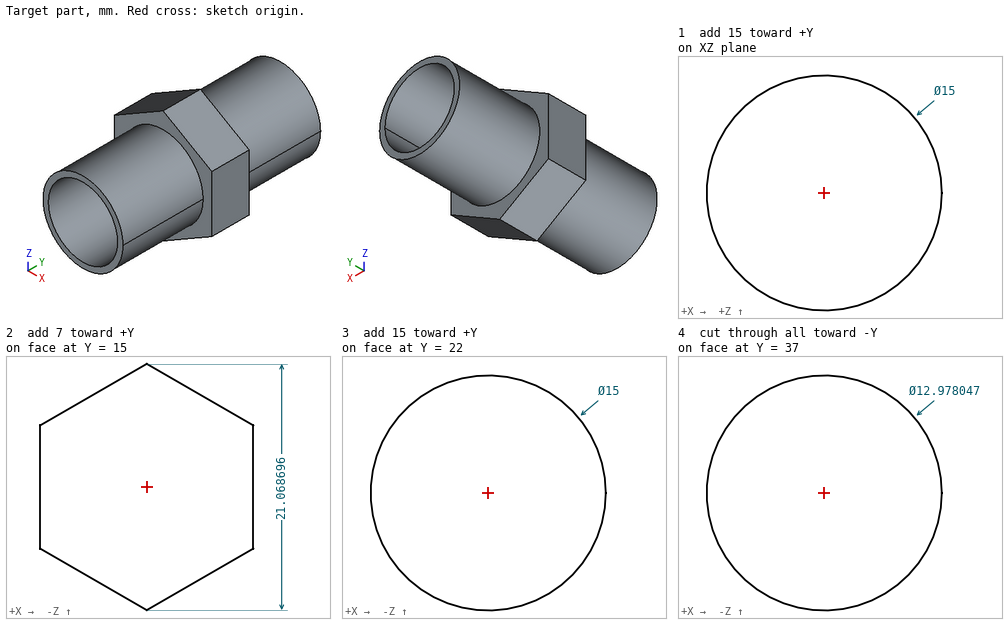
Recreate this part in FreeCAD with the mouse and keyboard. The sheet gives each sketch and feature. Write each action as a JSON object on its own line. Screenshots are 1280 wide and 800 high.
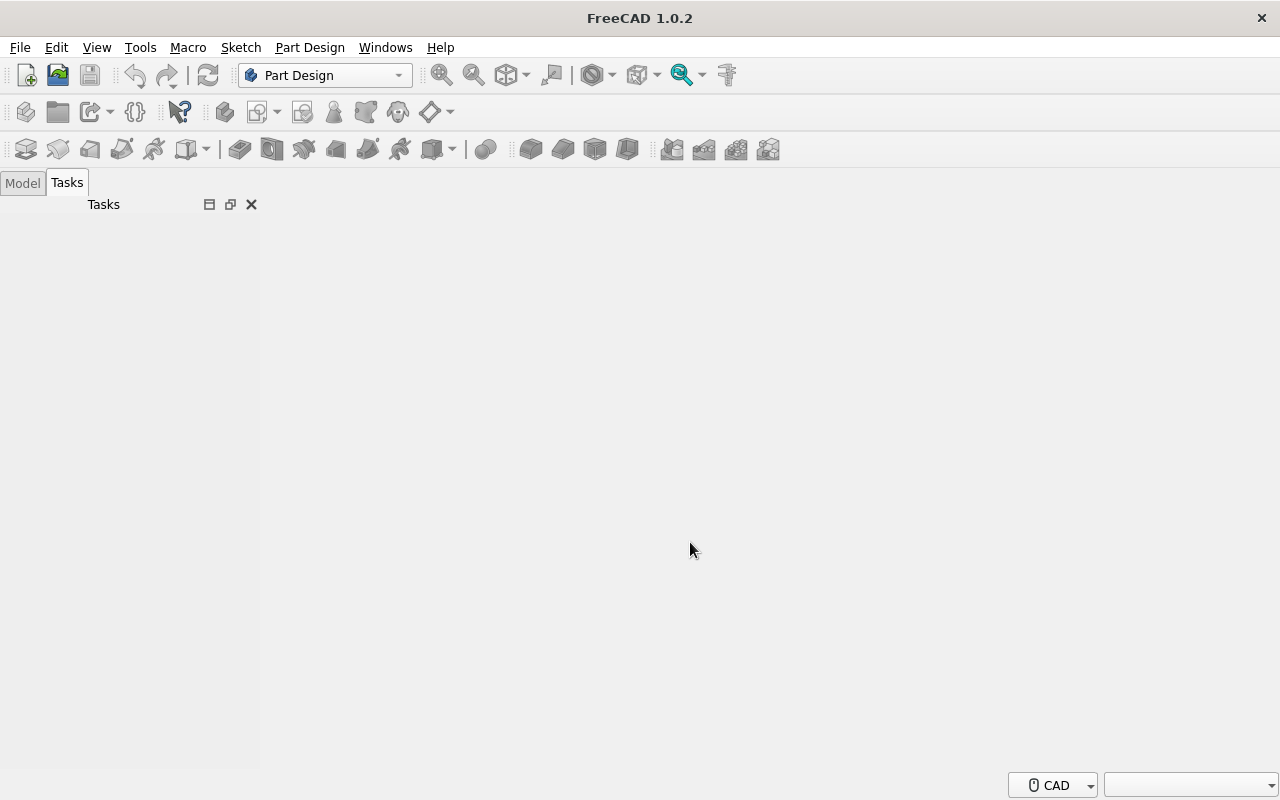
{"action": "left_click", "coordinate": [26, 76]}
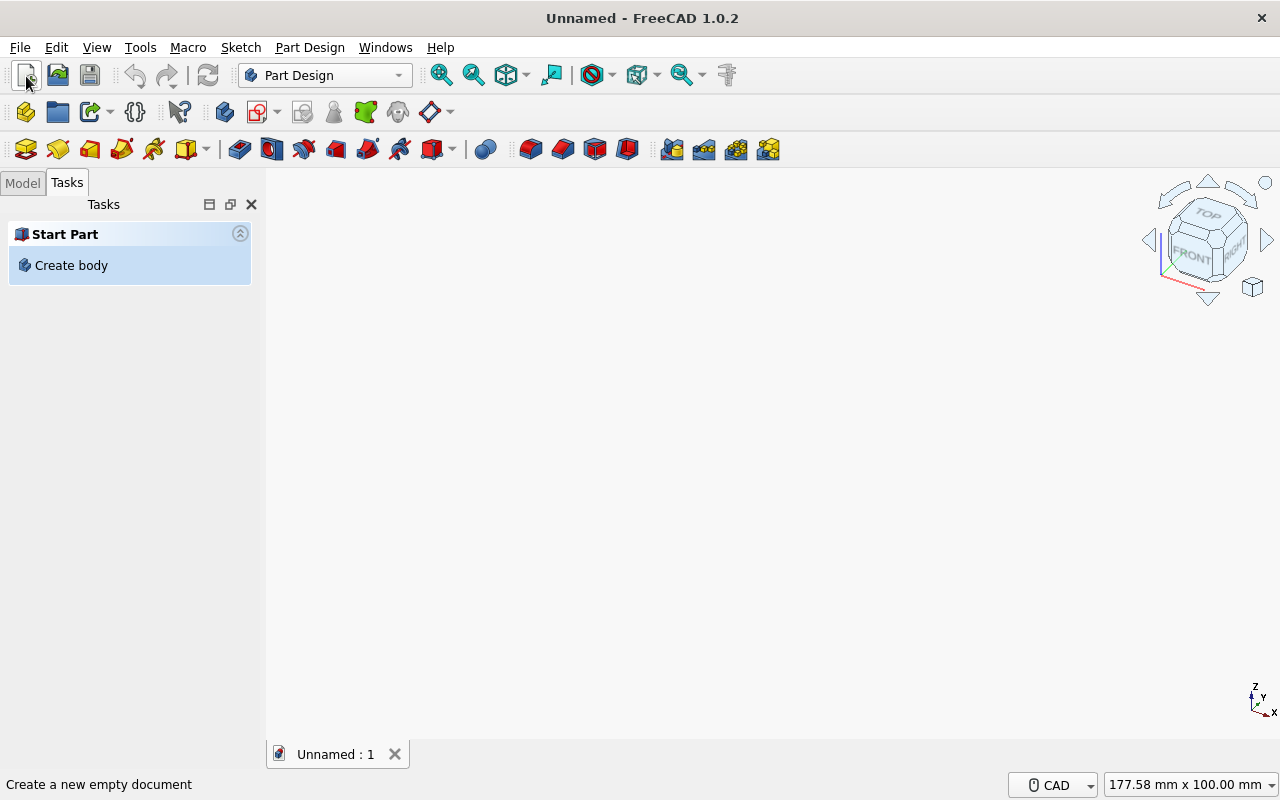
{"action": "left_click", "coordinate": [258, 112]}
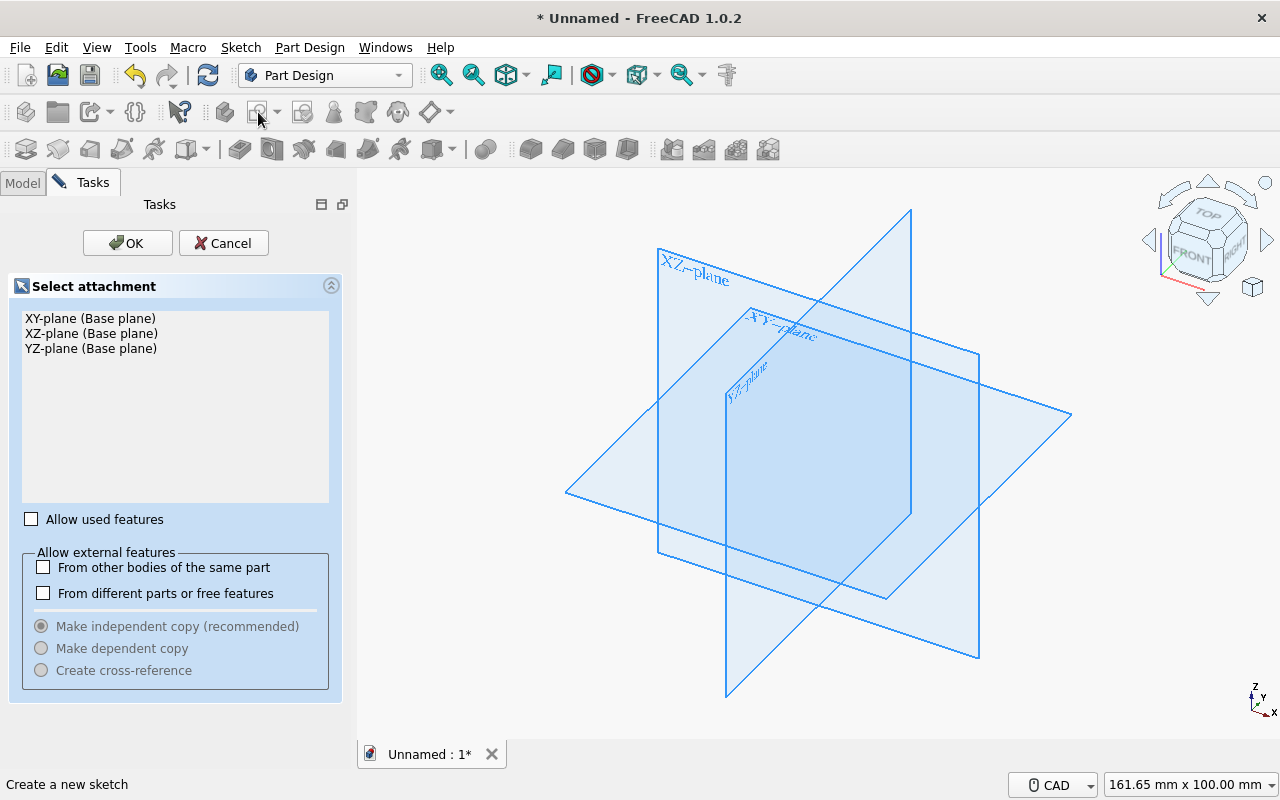
{"action": "left_click", "coordinate": [82, 334]}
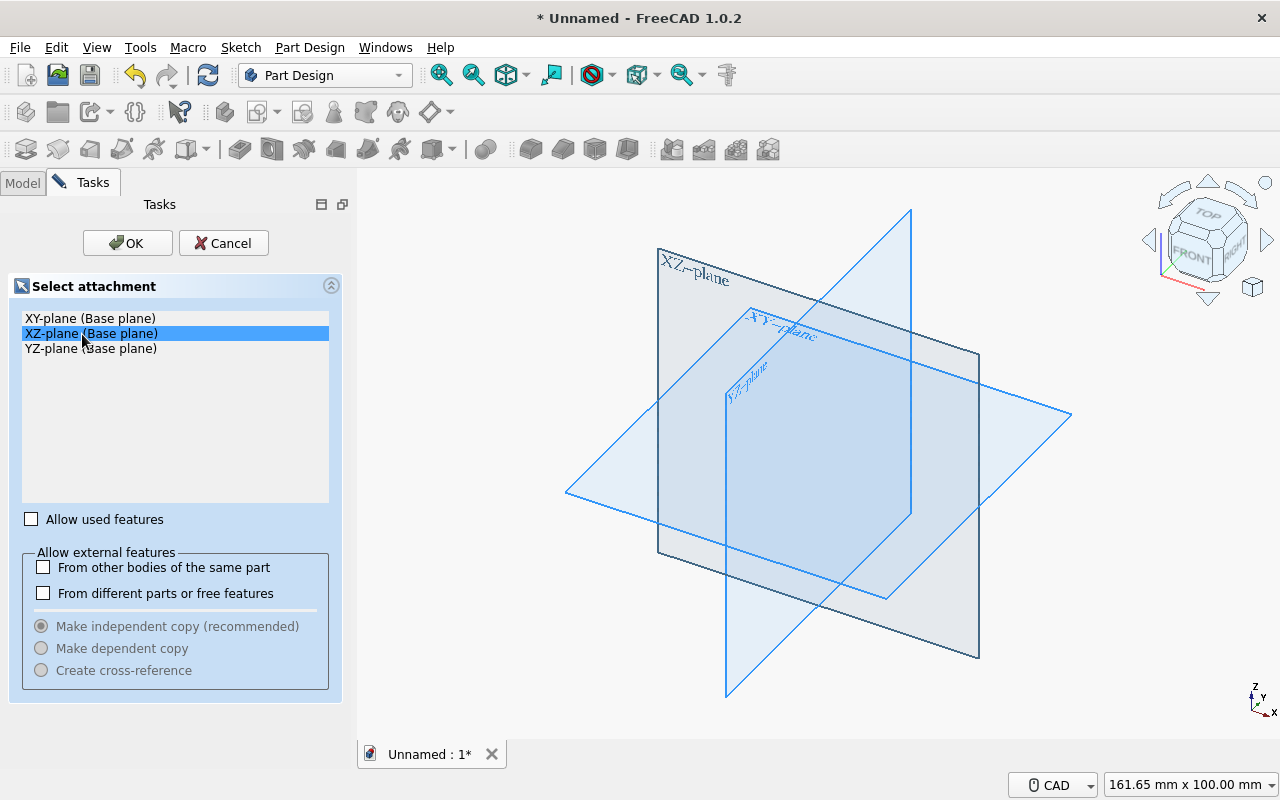
{"action": "left_click", "coordinate": [128, 243]}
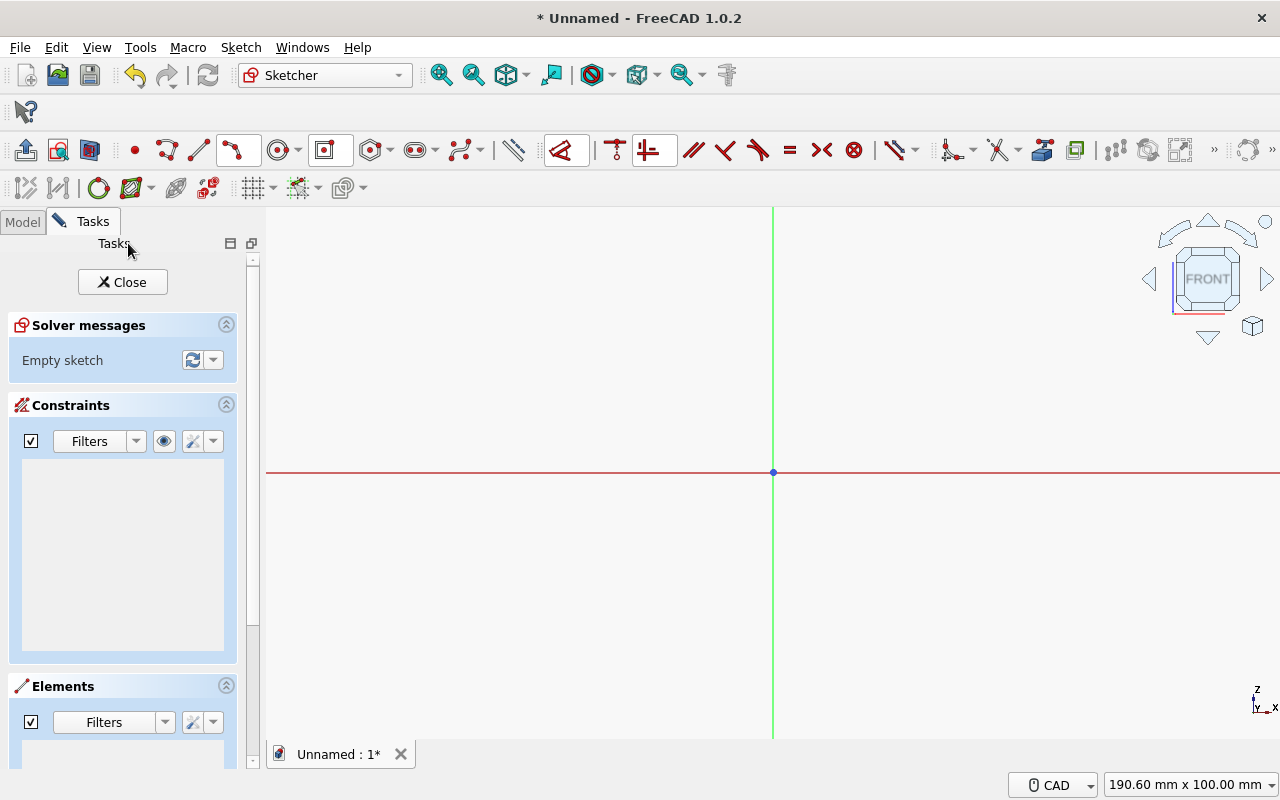
{"action": "scroll", "coordinate": [795, 473], "scroll_direction": "up", "scroll_amount": 7}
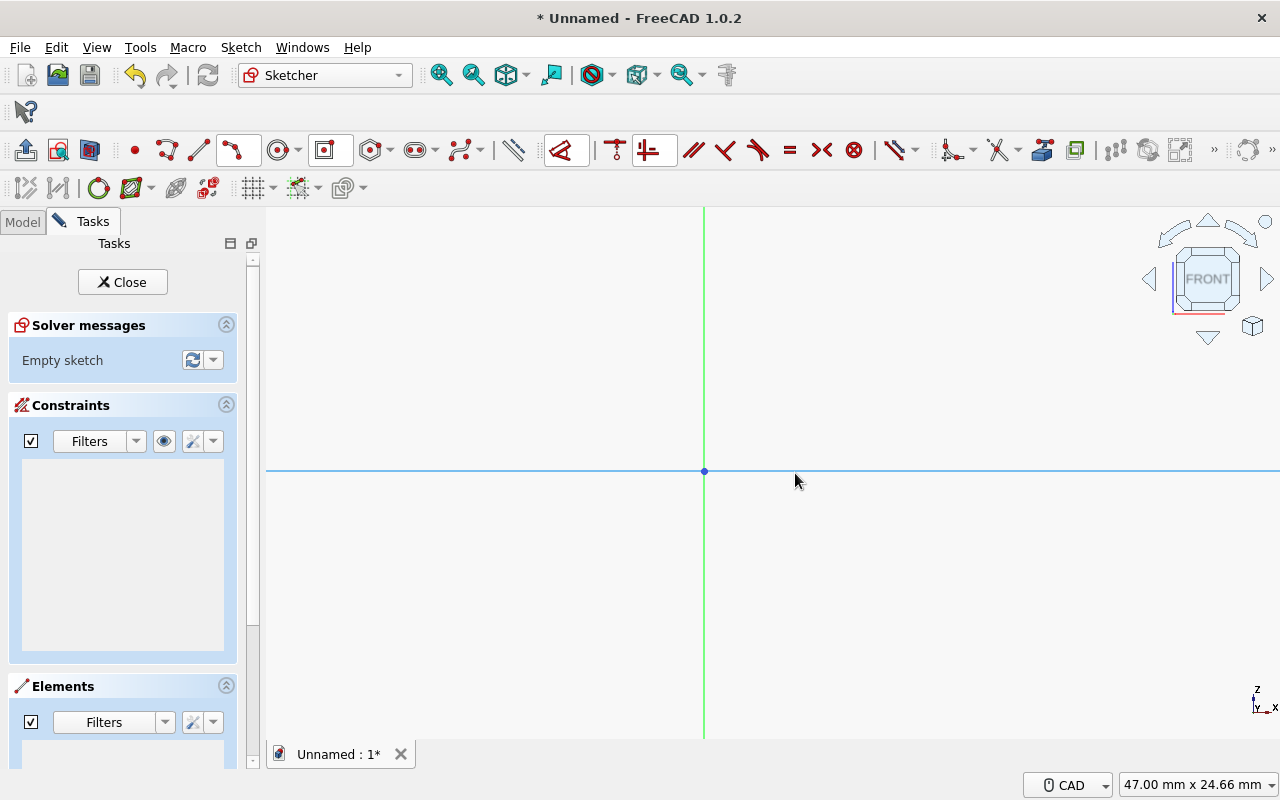
{"action": "left_click", "coordinate": [278, 150]}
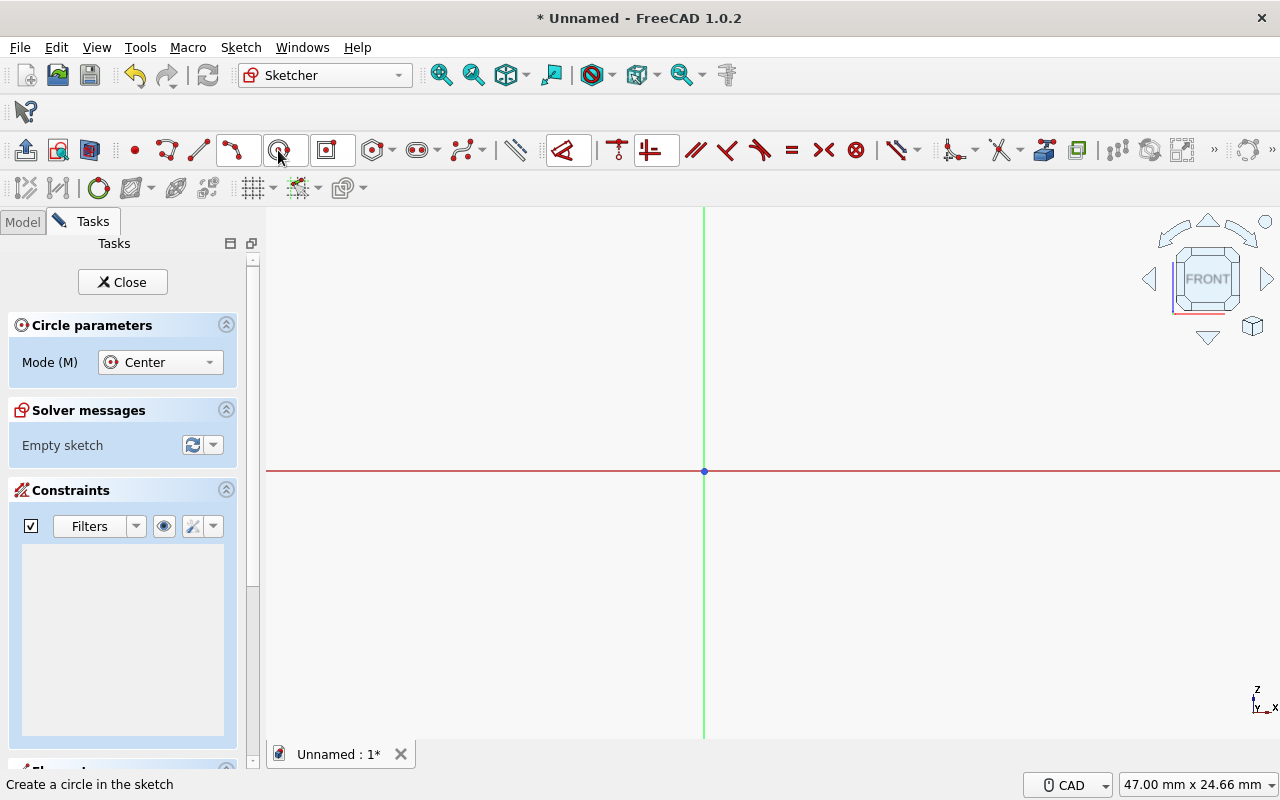
{"action": "left_click", "coordinate": [704, 471]}
{"action": "mouse_move", "coordinate": [819, 357]}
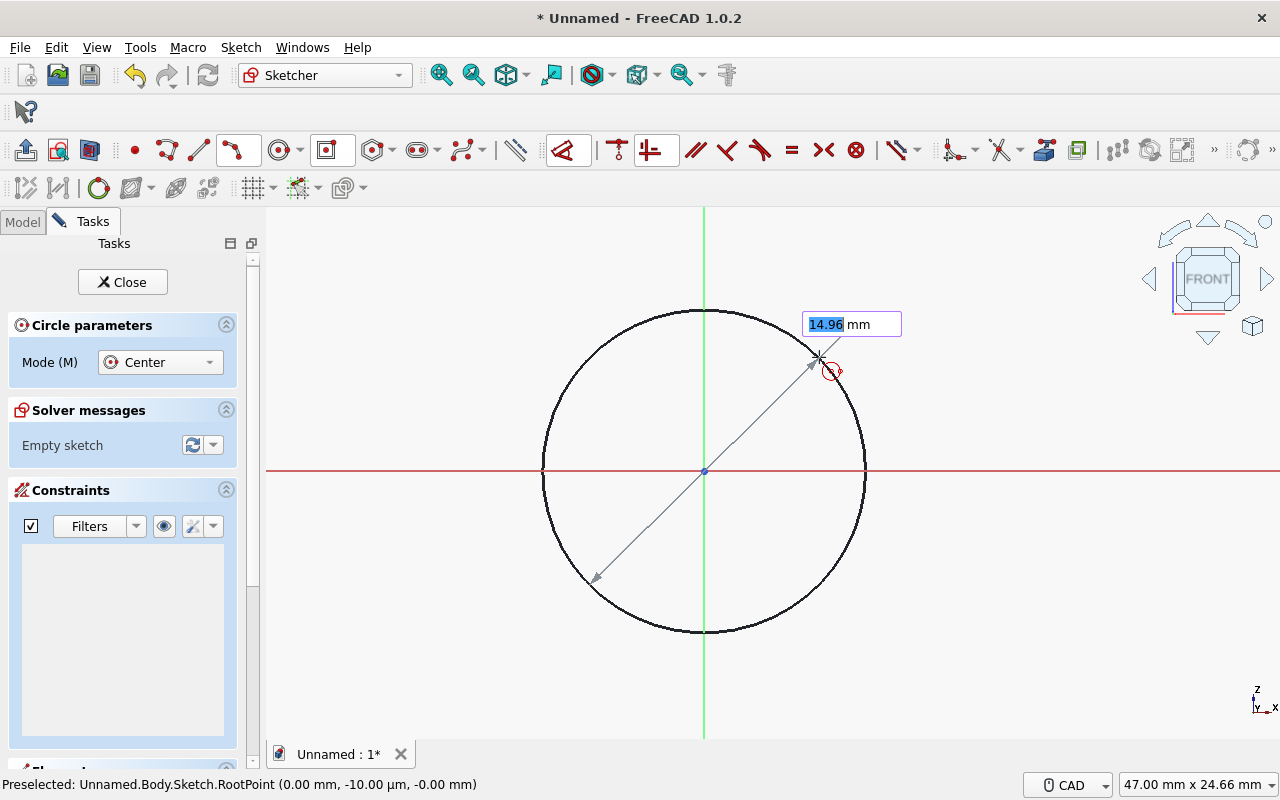
{"action": "type", "text": "15"}
{"action": "key", "text": "Return"}
{"action": "key", "text": "Escape"}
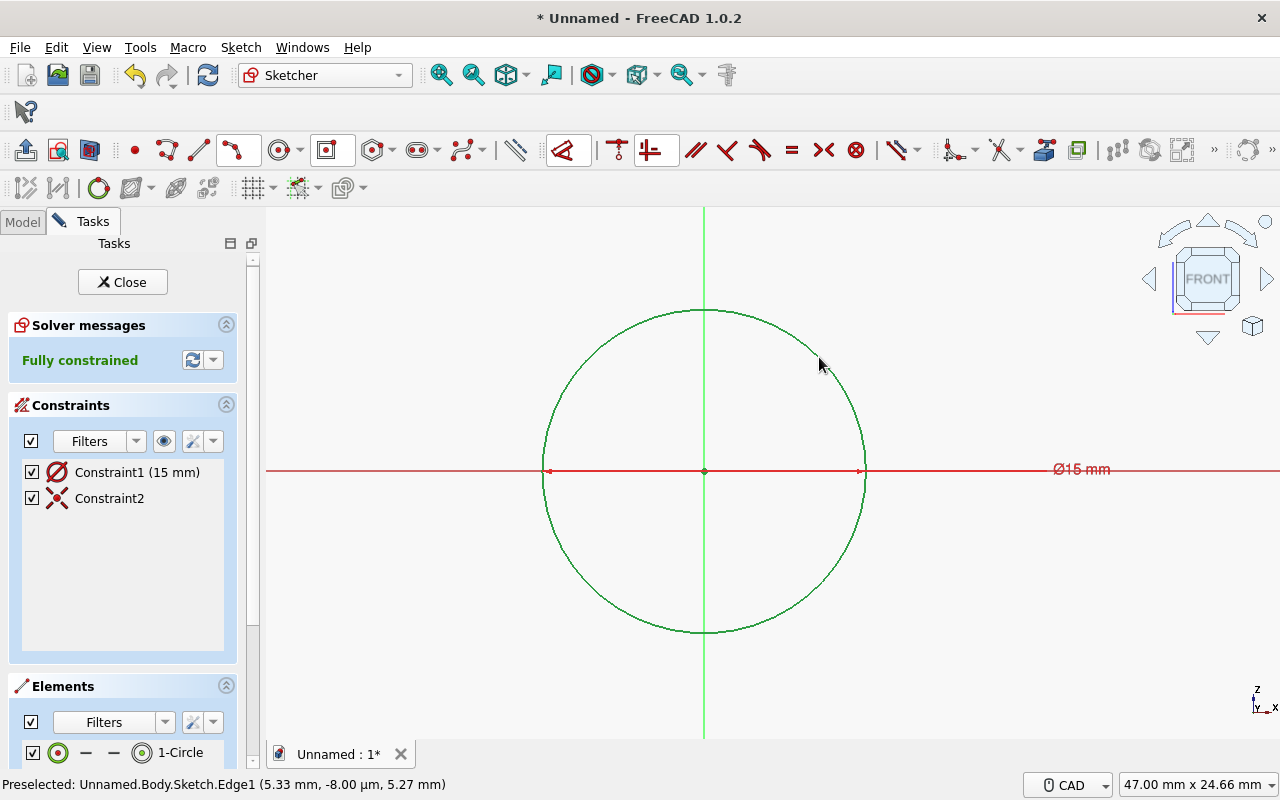
{"action": "left_click", "coordinate": [123, 282]}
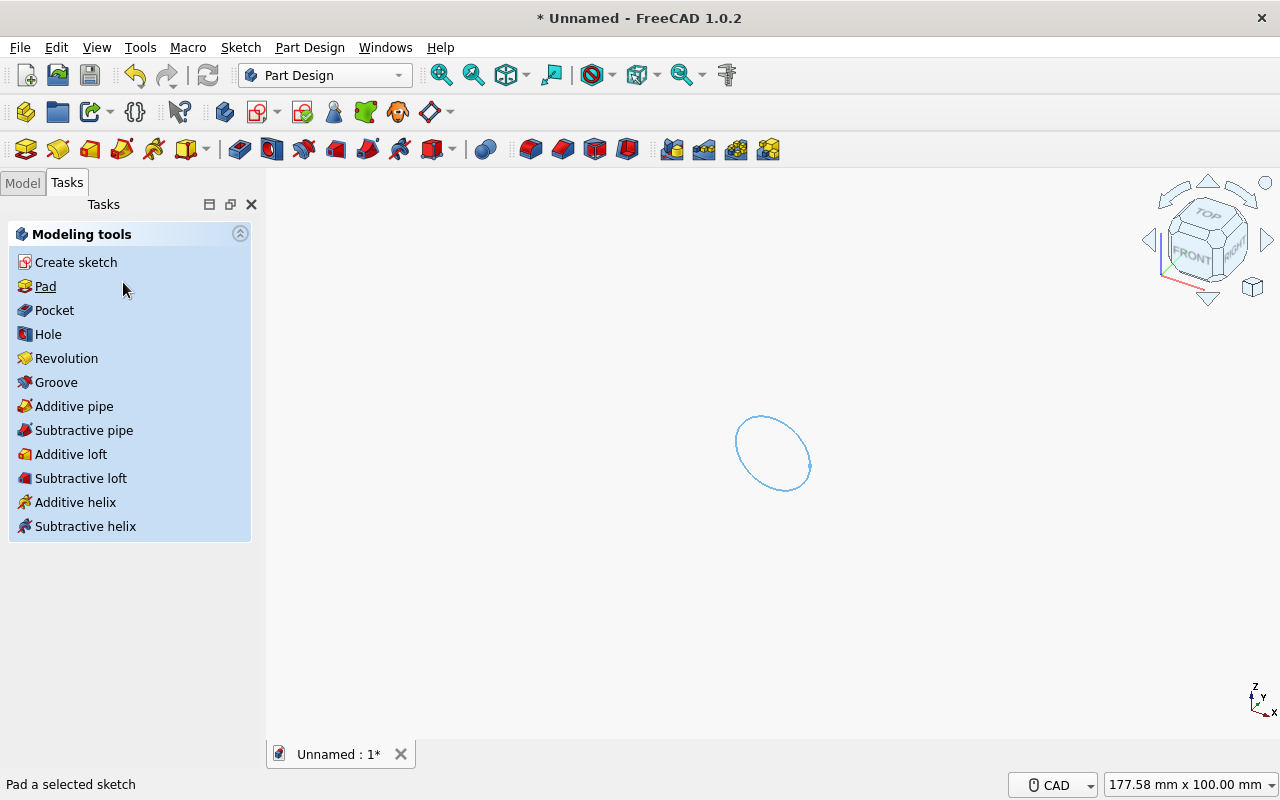
{"action": "left_click", "coordinate": [26, 150]}